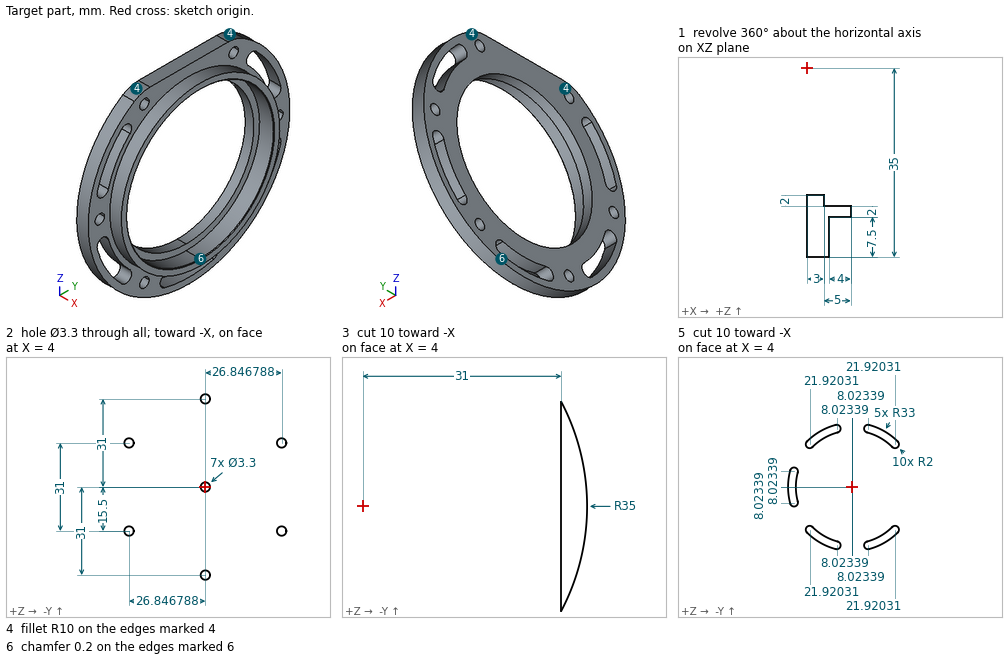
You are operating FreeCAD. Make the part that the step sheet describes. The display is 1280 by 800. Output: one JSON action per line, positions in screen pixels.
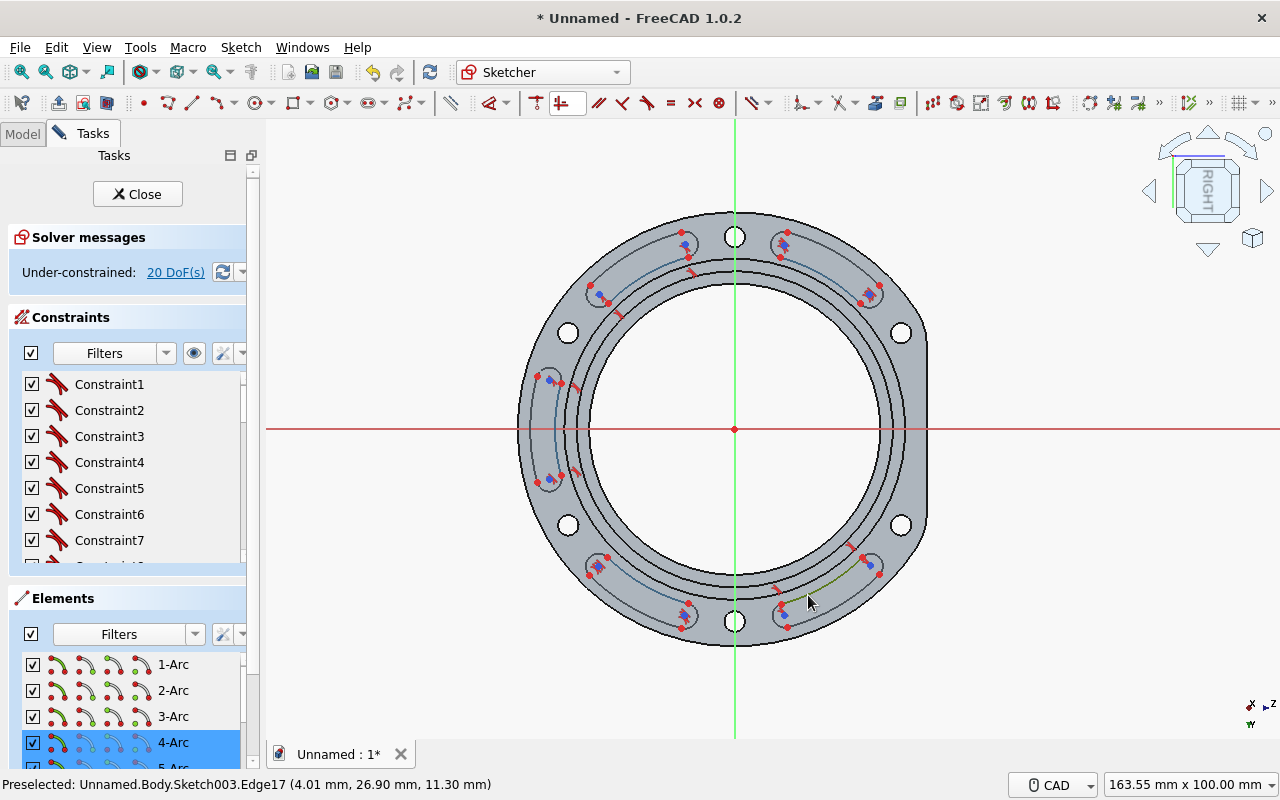
{"action": "left_click", "coordinate": [672, 104]}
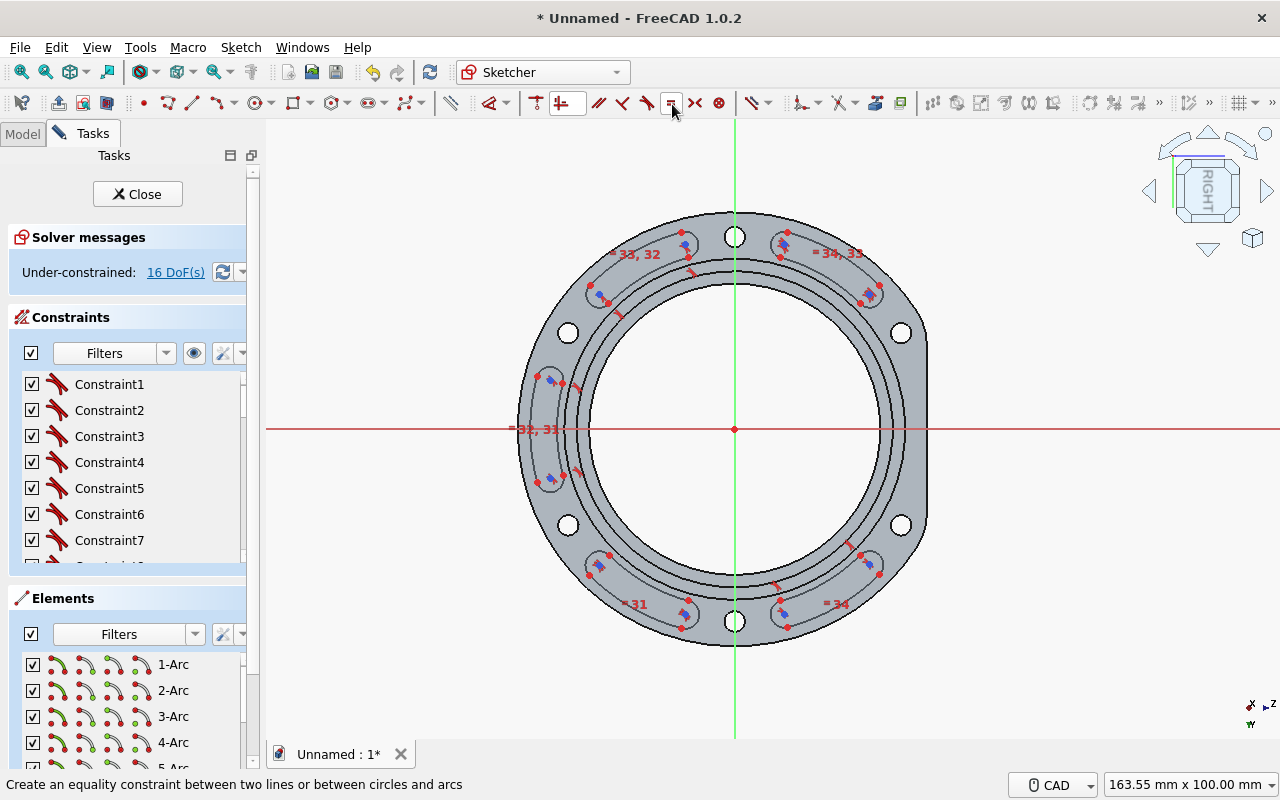
{"action": "left_click", "coordinate": [597, 551]}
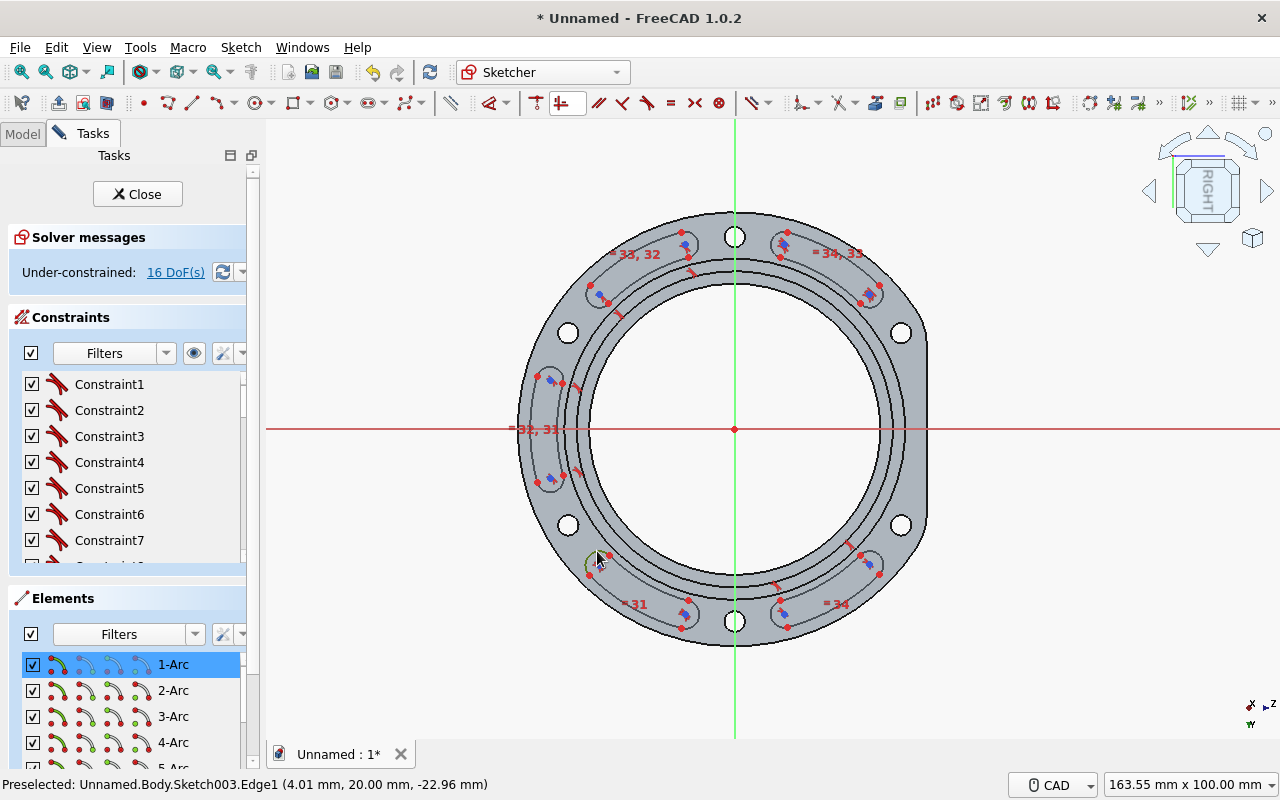
{"action": "left_click", "coordinate": [560, 372]}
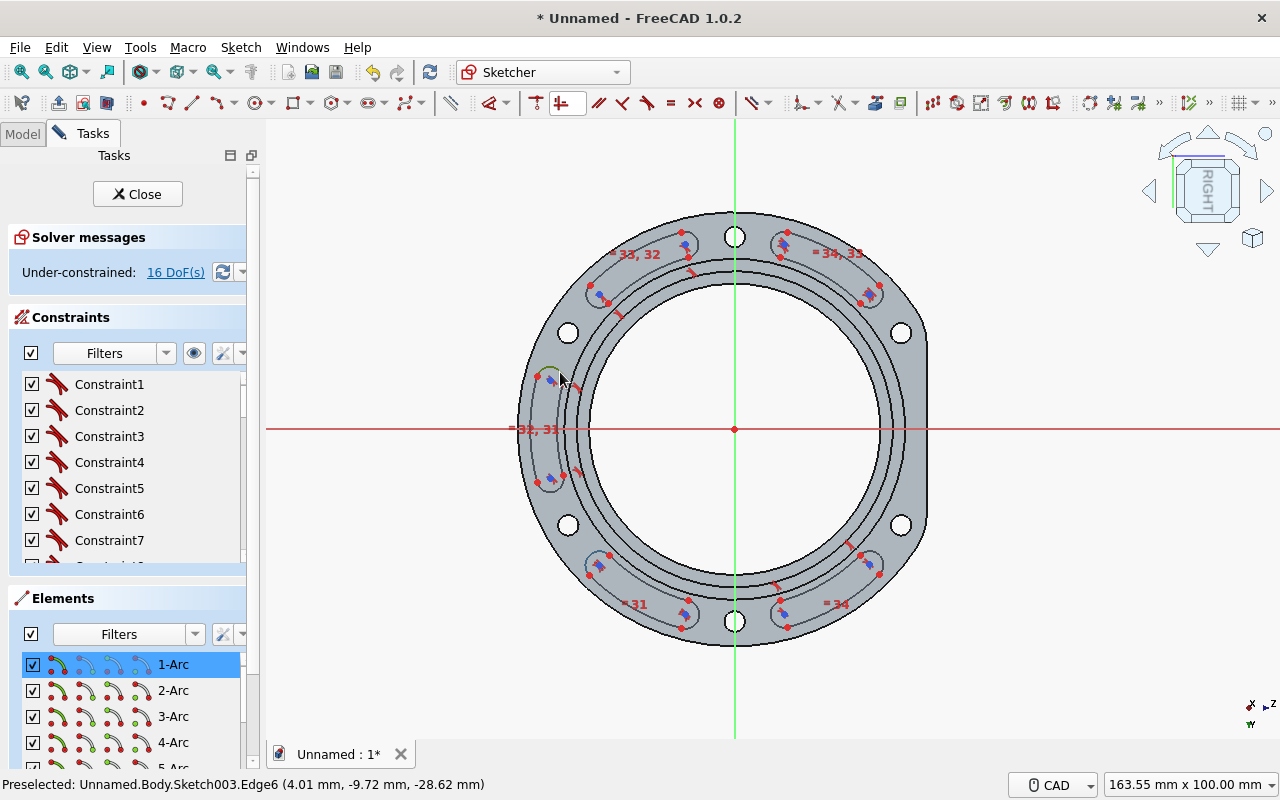
{"action": "left_click", "coordinate": [698, 250]}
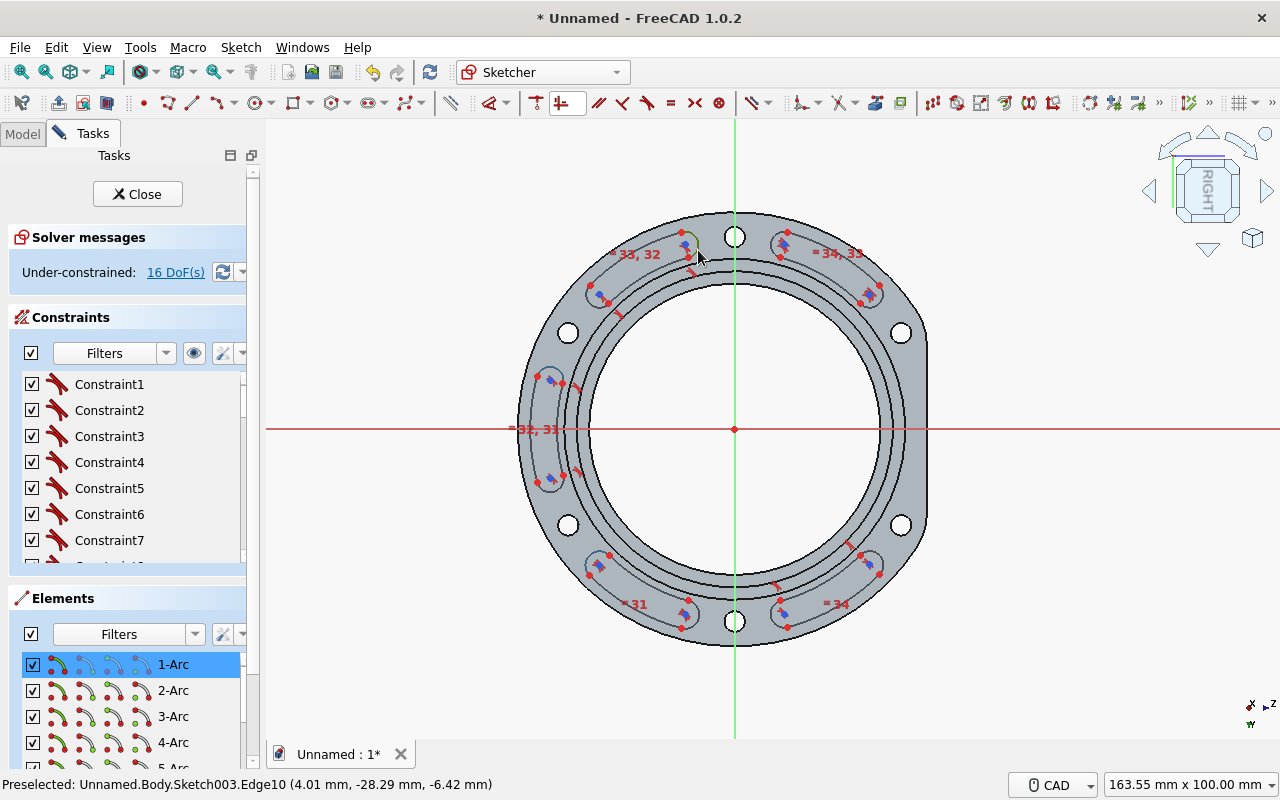
{"action": "left_click", "coordinate": [872, 307]}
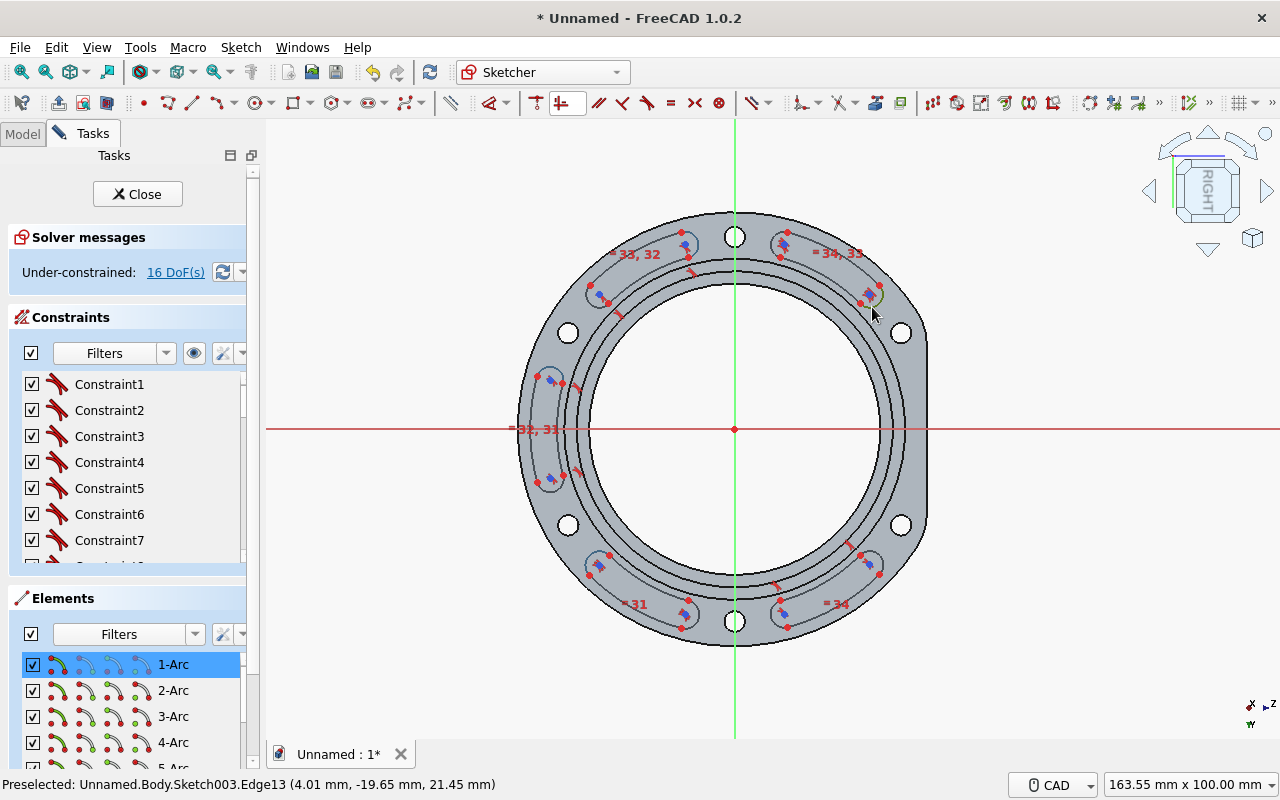
{"action": "left_click", "coordinate": [772, 609]}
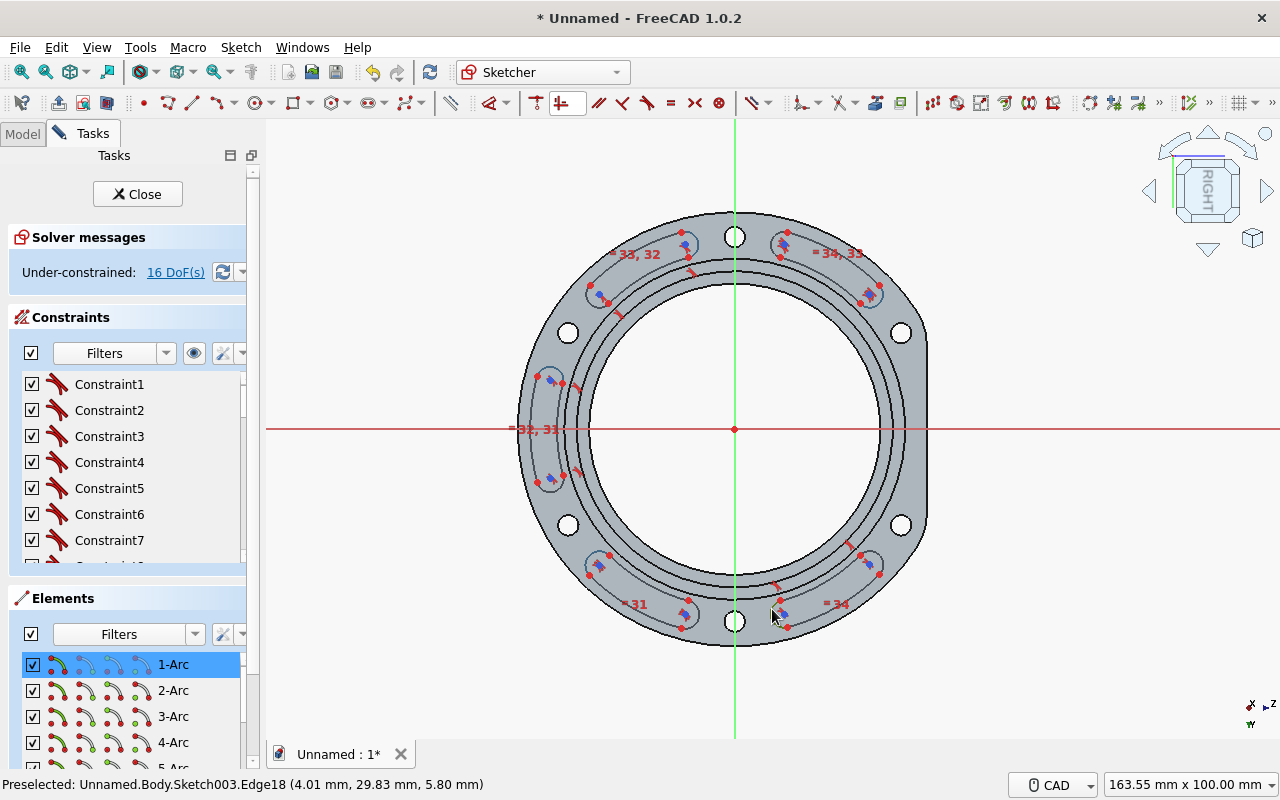
{"action": "left_click", "coordinate": [672, 104]}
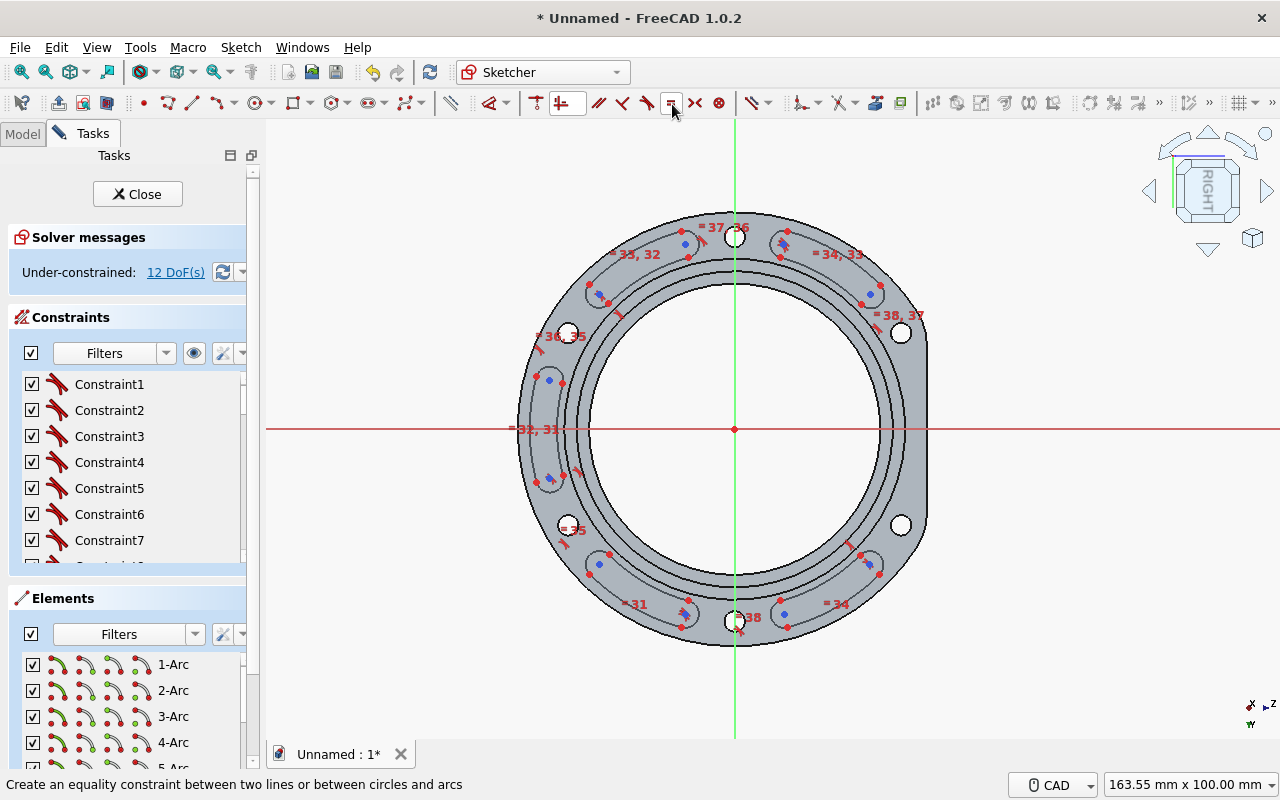
{"action": "left_click", "coordinate": [490, 104]}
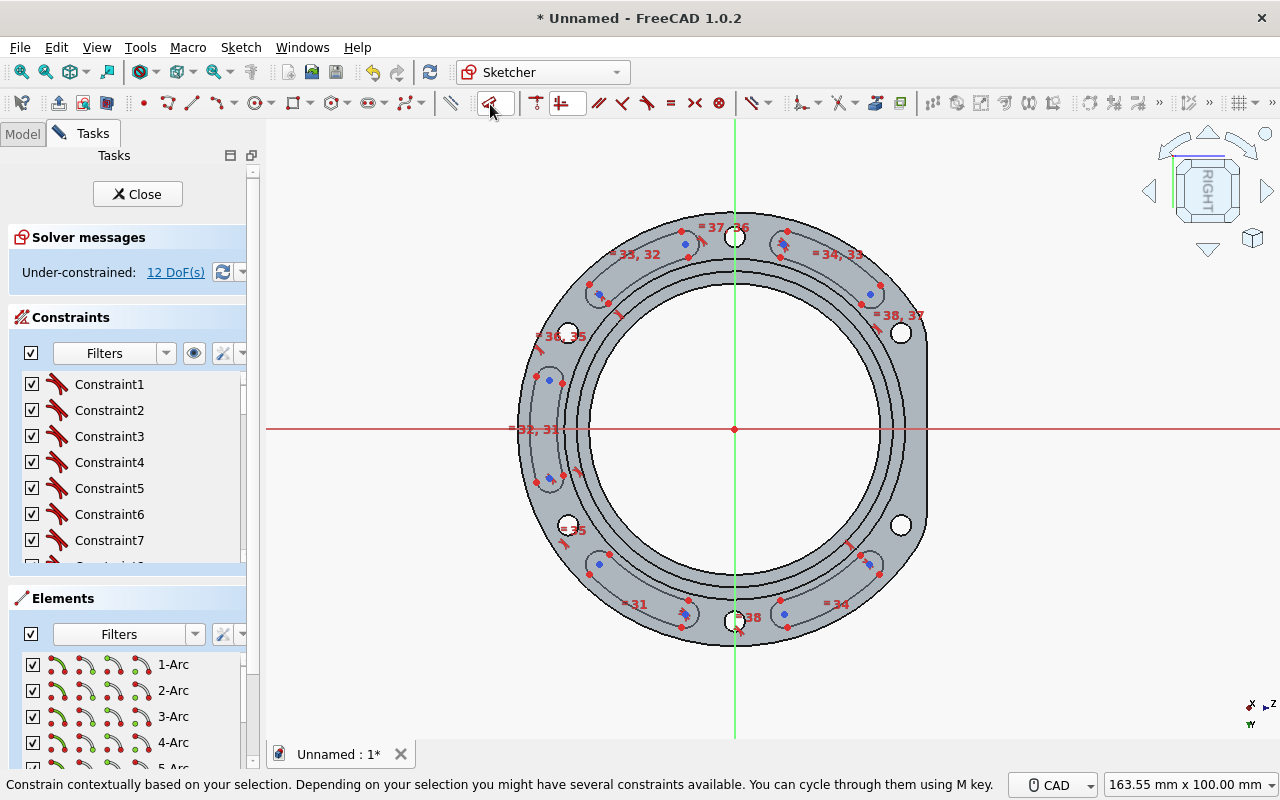
{"action": "scroll", "coordinate": [597, 551], "scroll_direction": "up", "scroll_amount": 6}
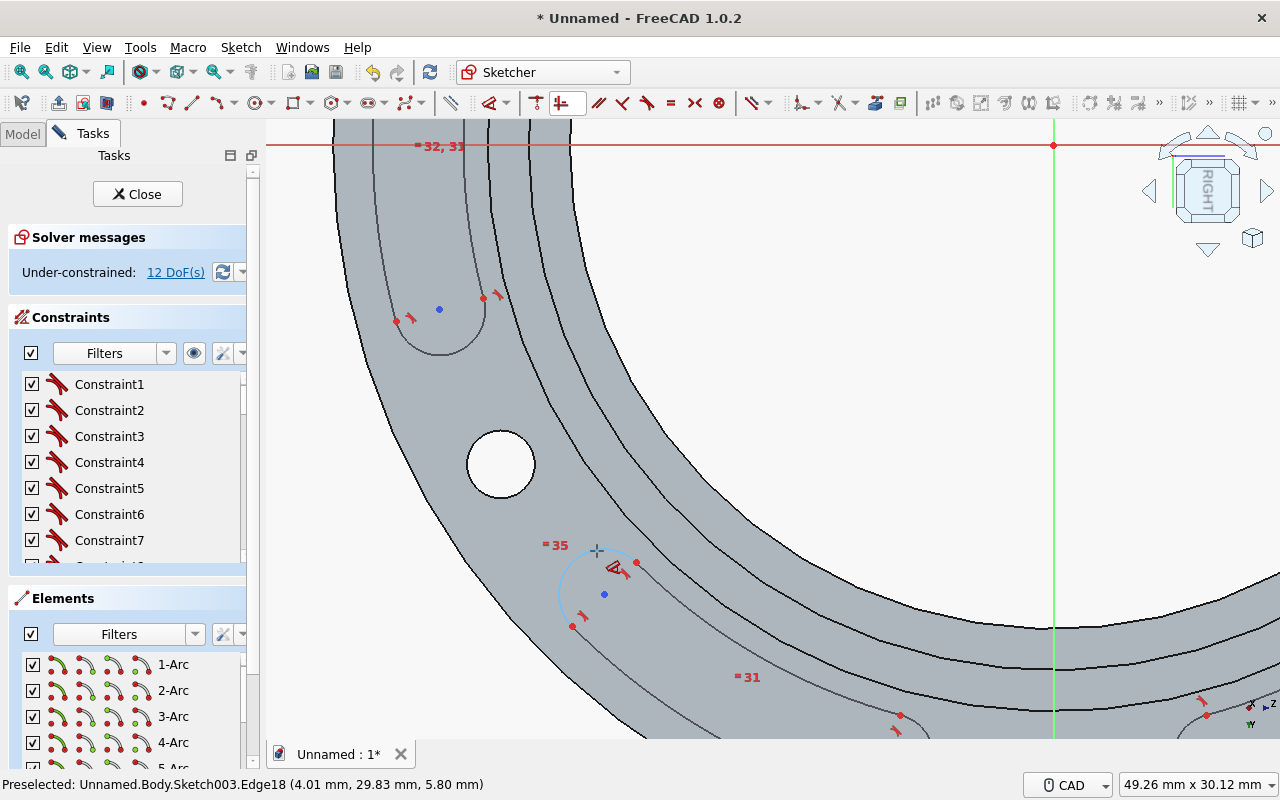
{"action": "left_click", "coordinate": [597, 550]}
{"action": "left_click", "coordinate": [592, 518]}